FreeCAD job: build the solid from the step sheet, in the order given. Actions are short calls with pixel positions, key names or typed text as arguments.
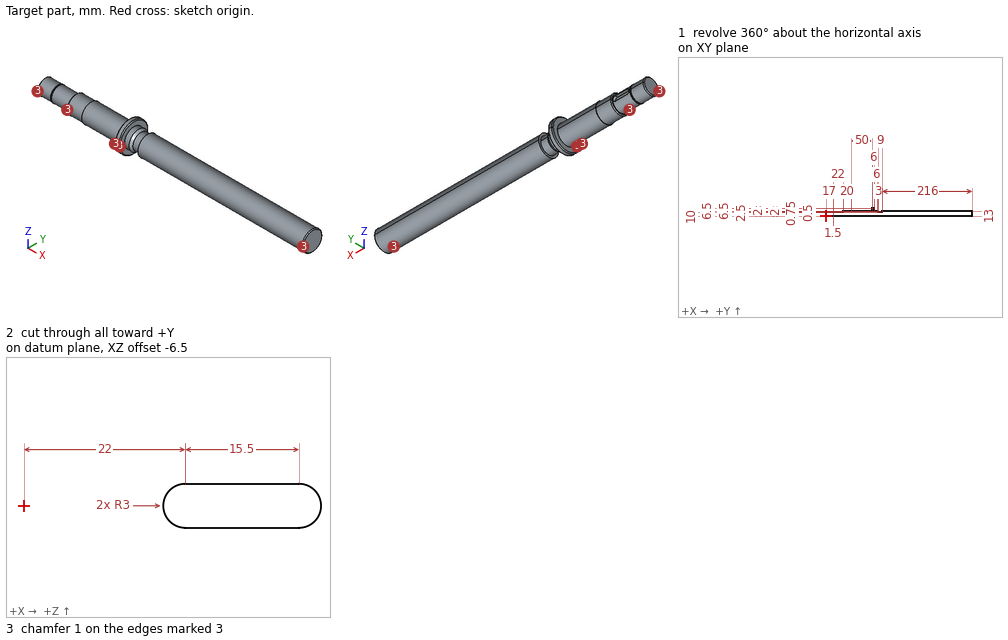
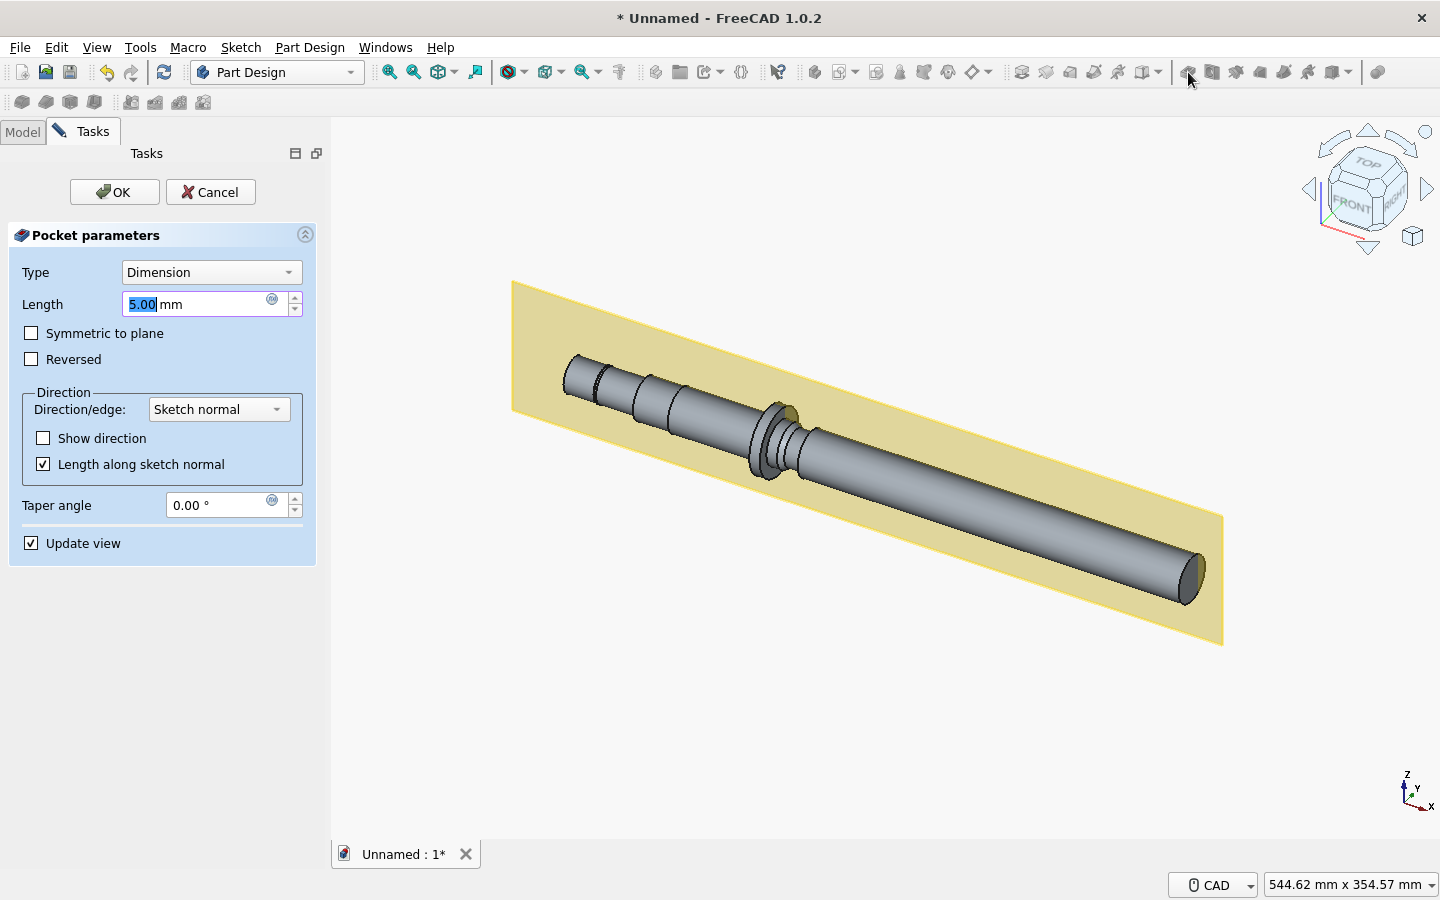
click(212, 272)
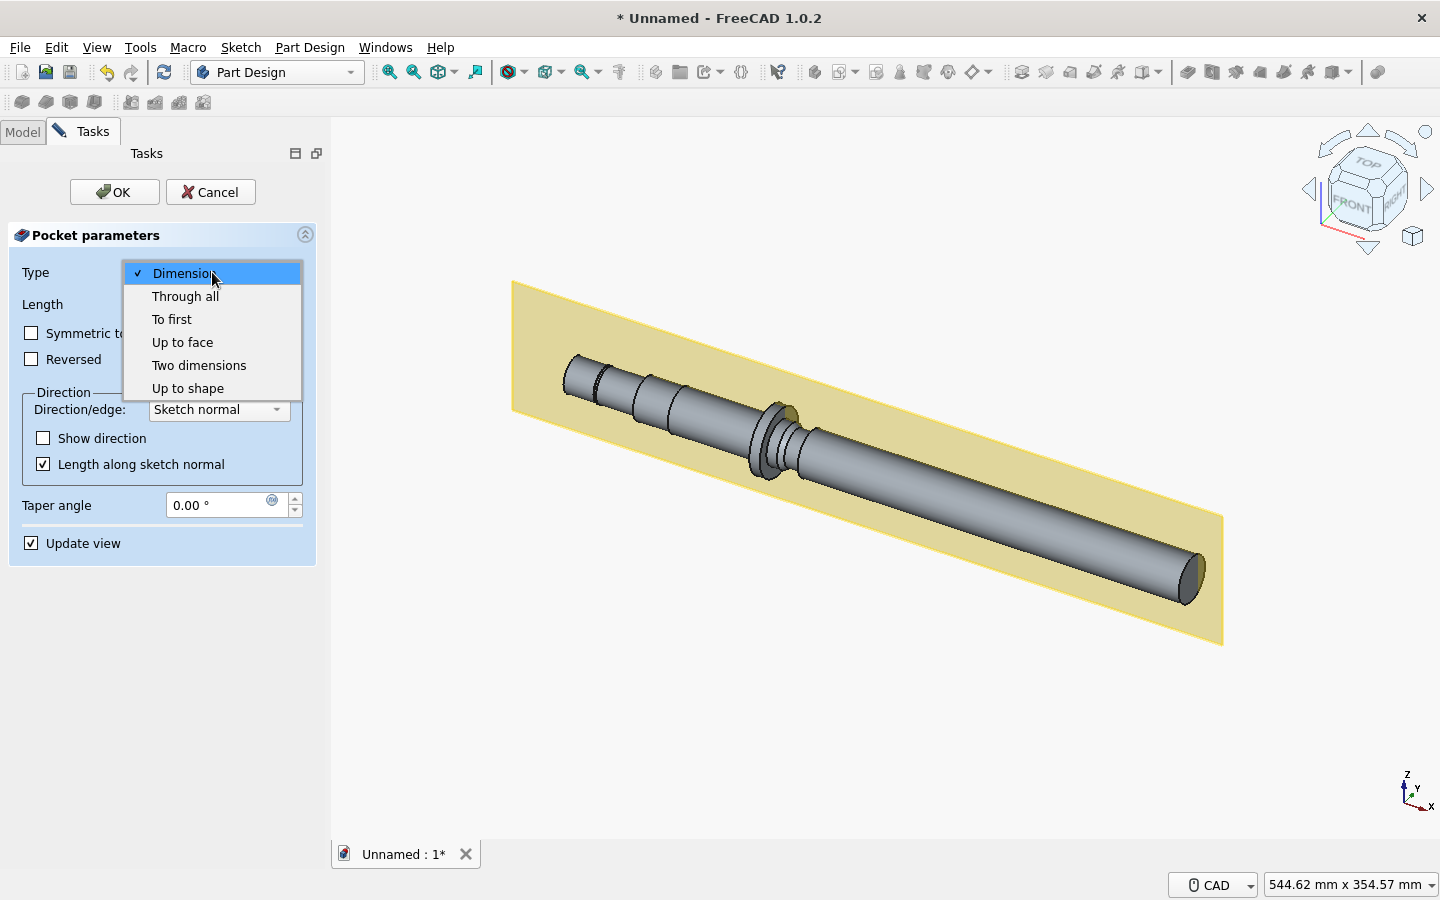
click(212, 296)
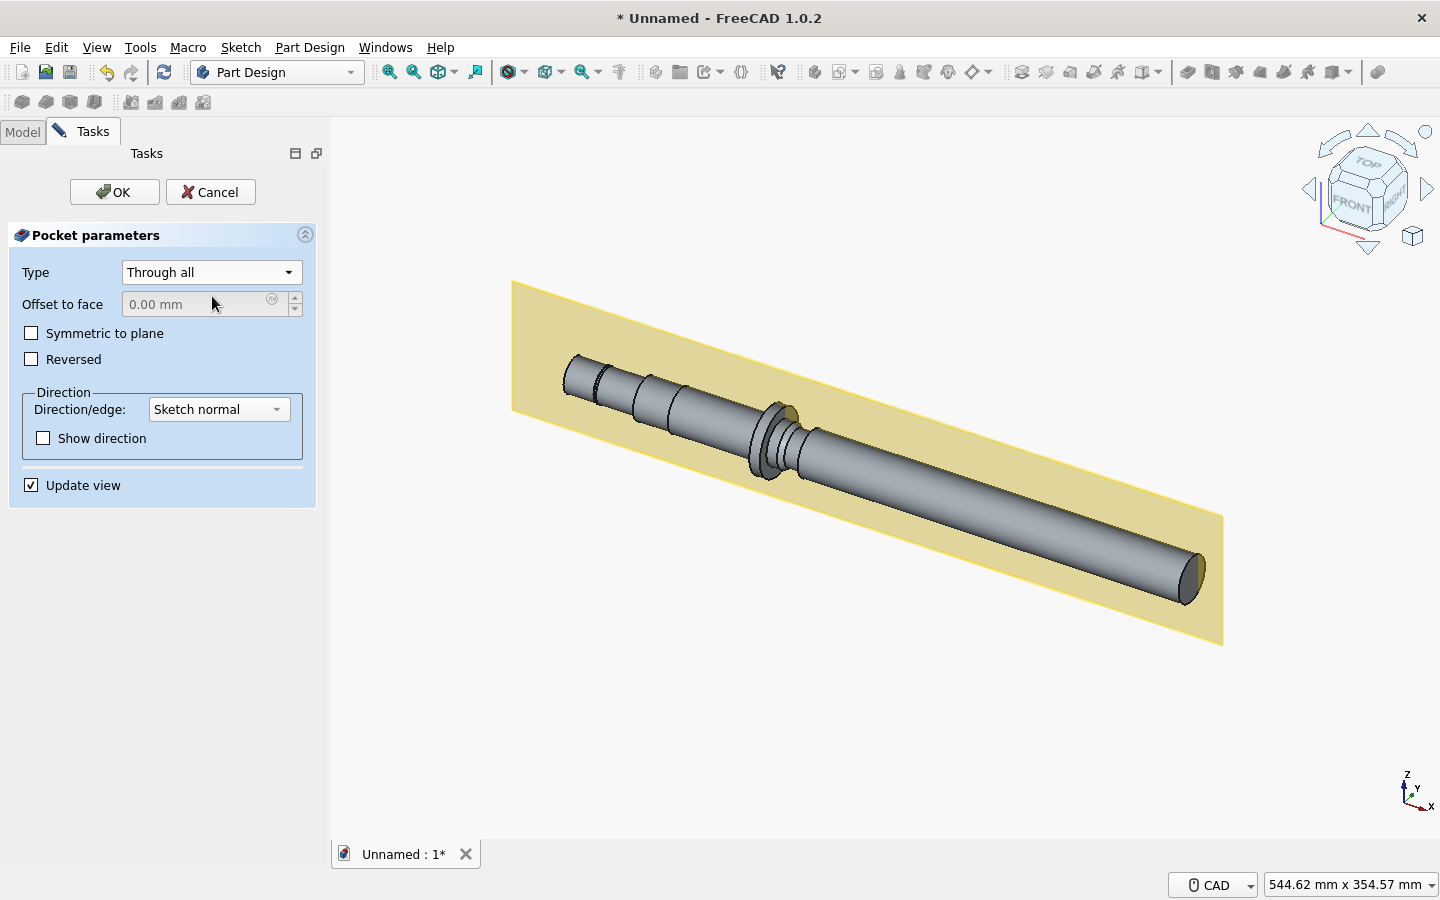
click(115, 192)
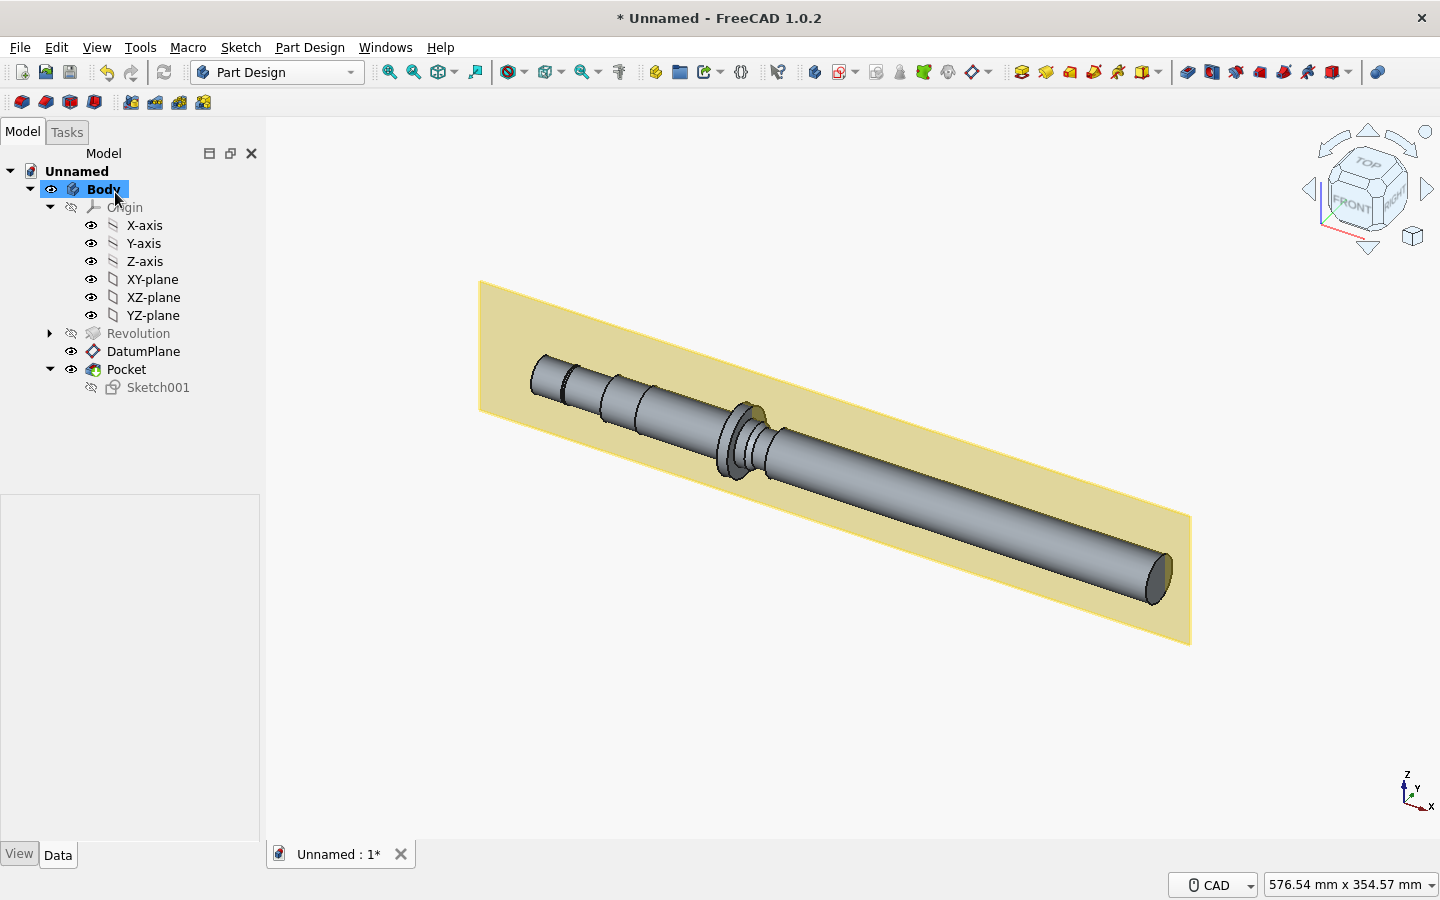
click(116, 351)
key(space)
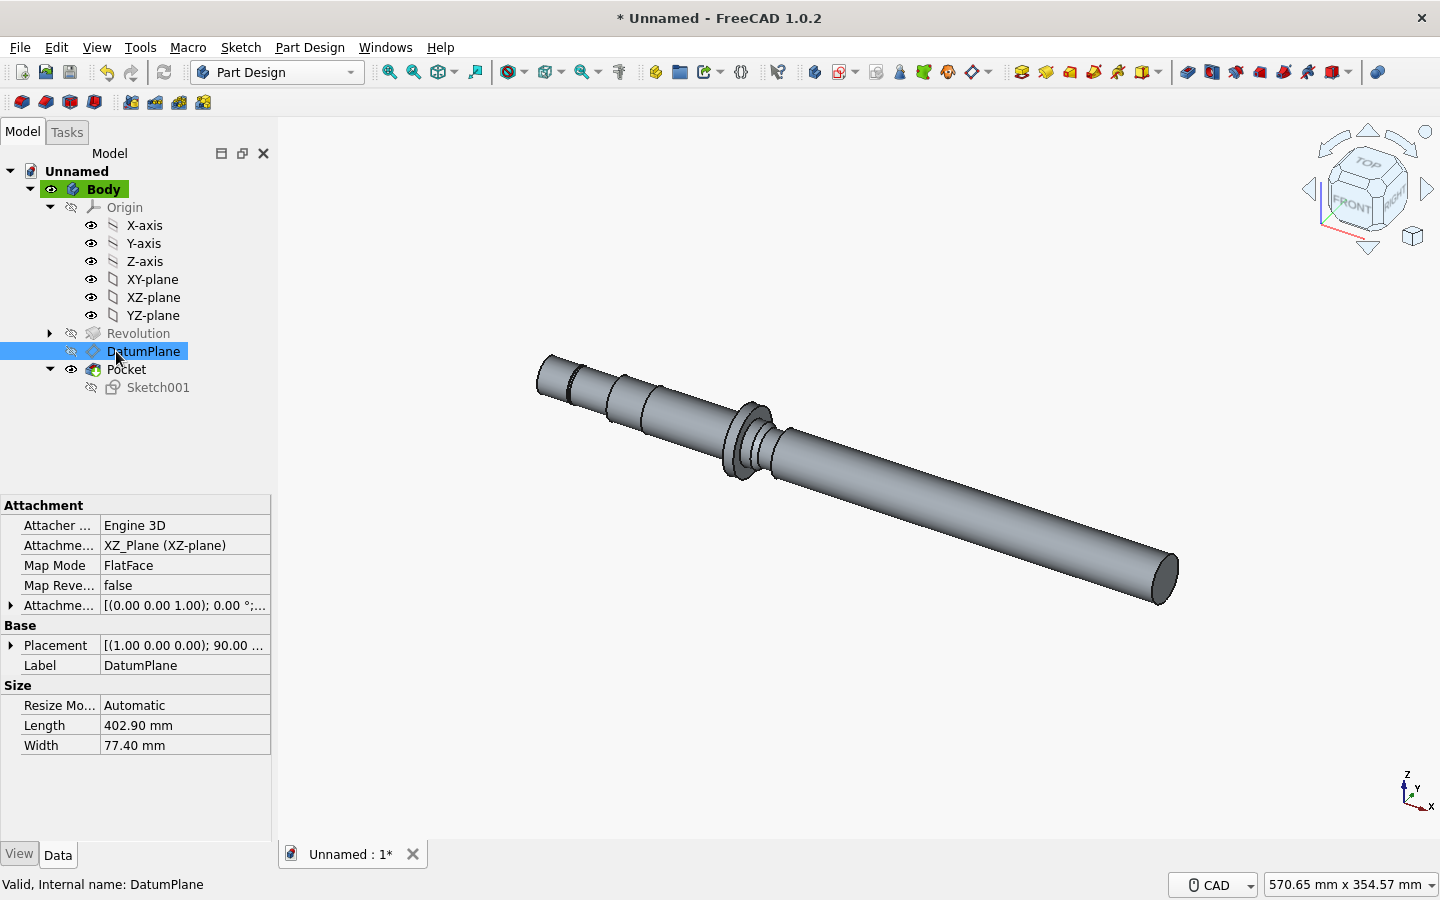
click(1152, 592)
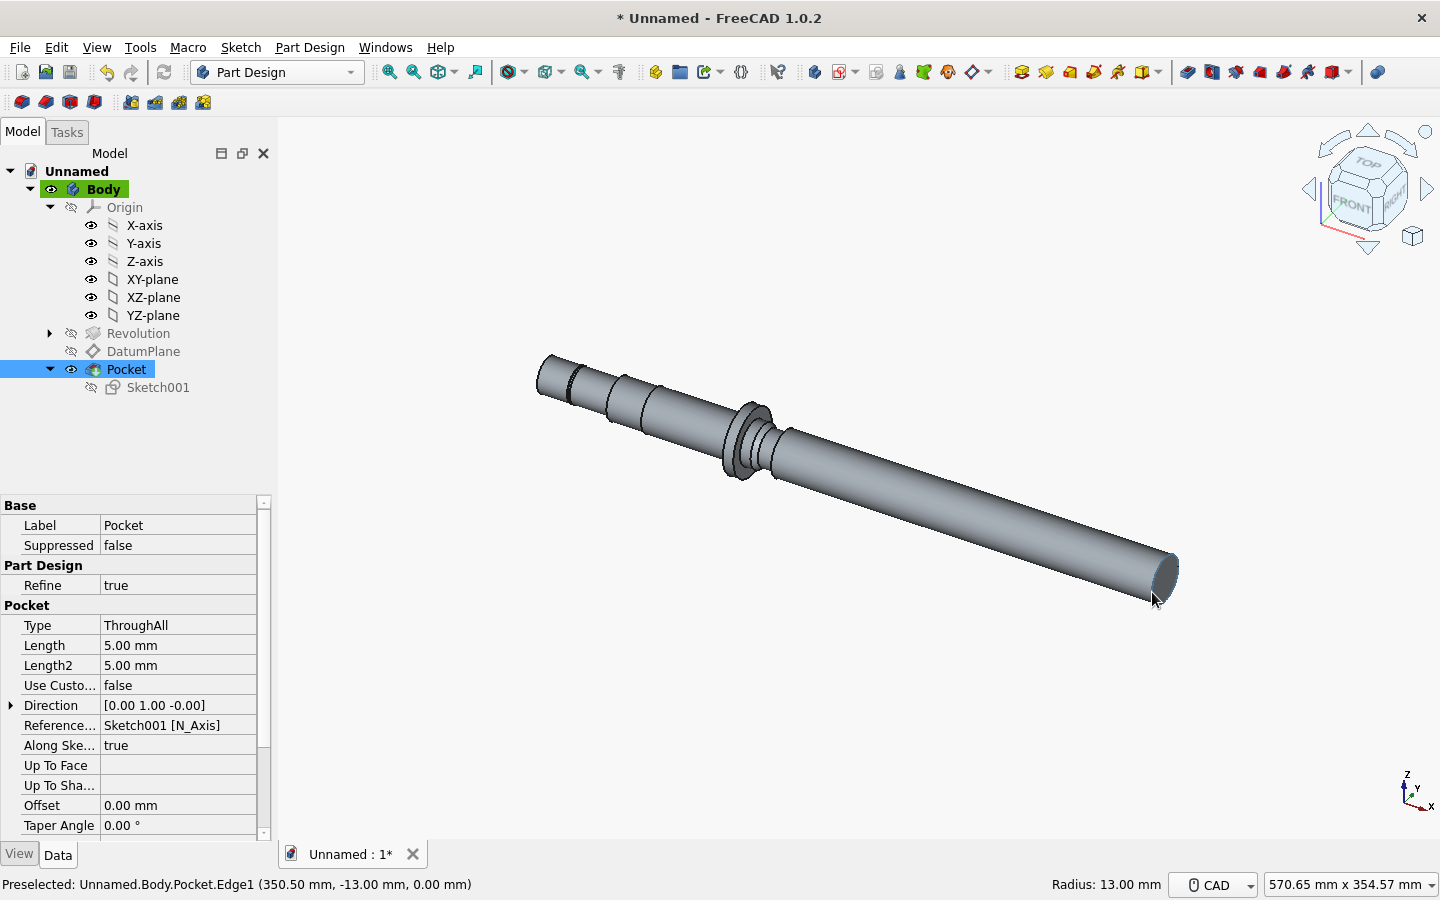
click(733, 461, ctrl)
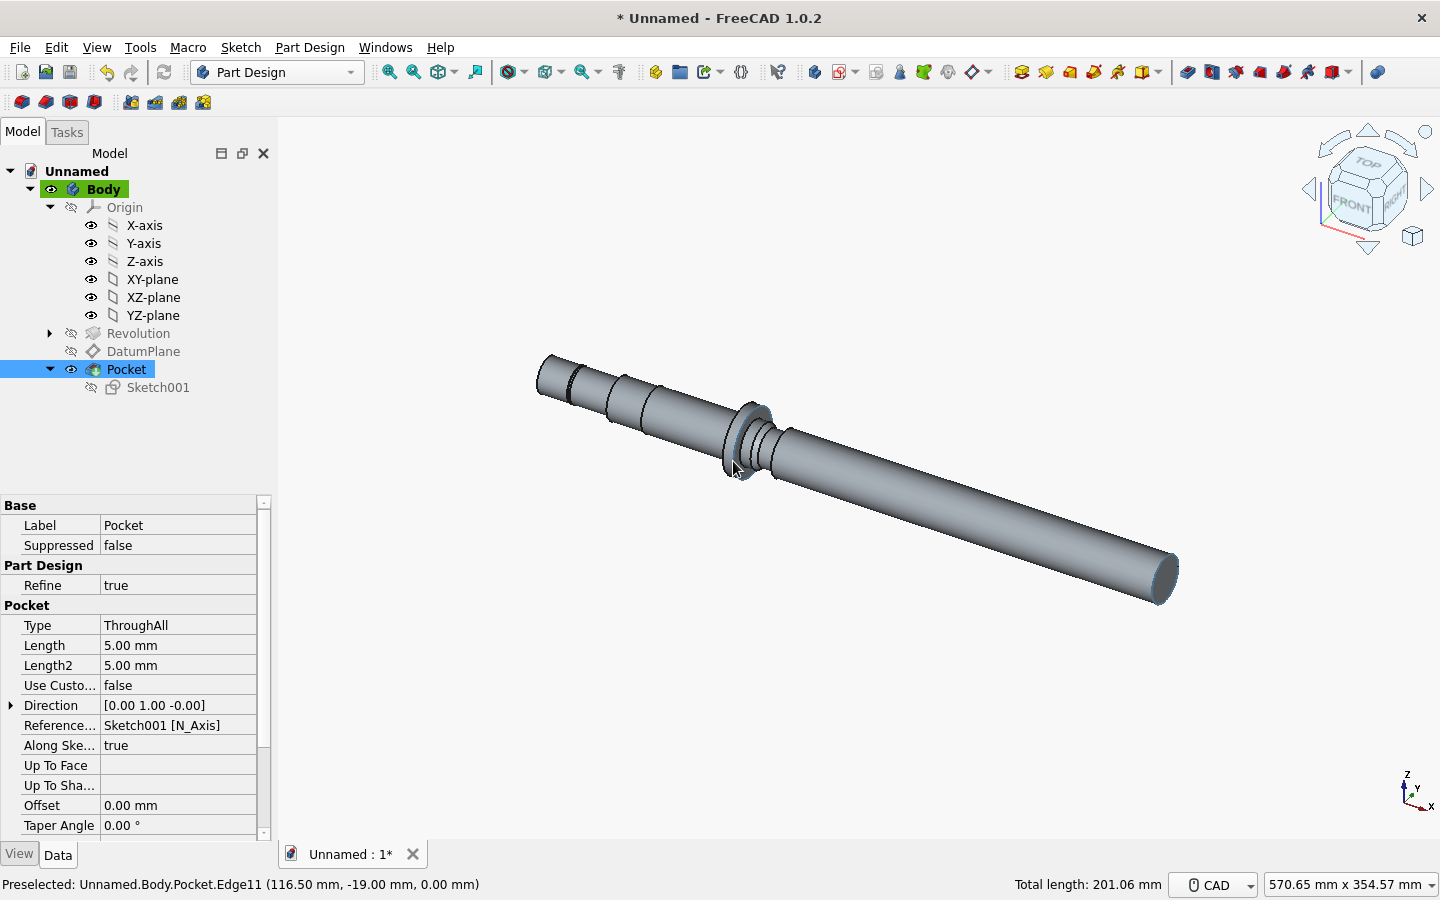
click(736, 414, ctrl)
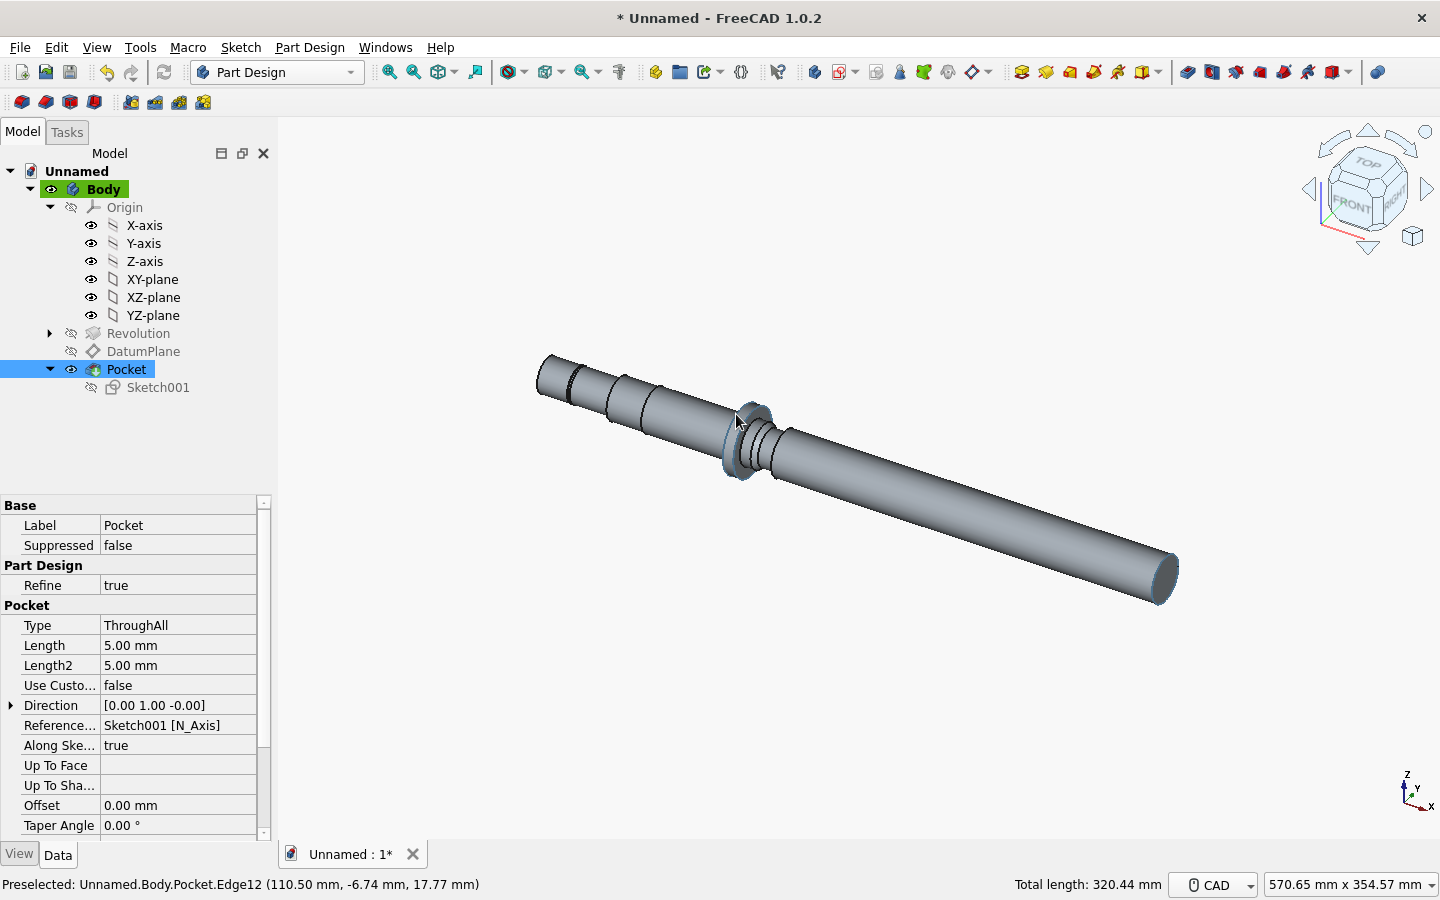
click(606, 410, ctrl)